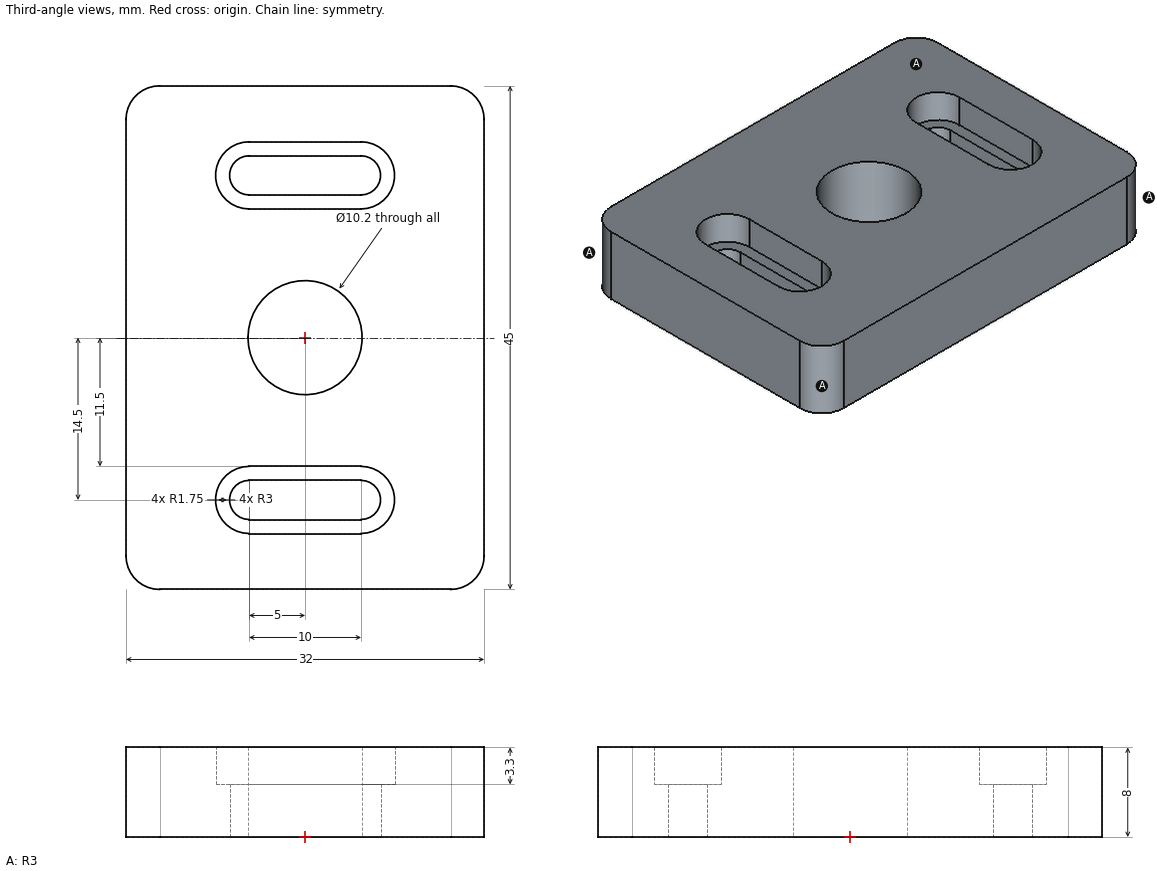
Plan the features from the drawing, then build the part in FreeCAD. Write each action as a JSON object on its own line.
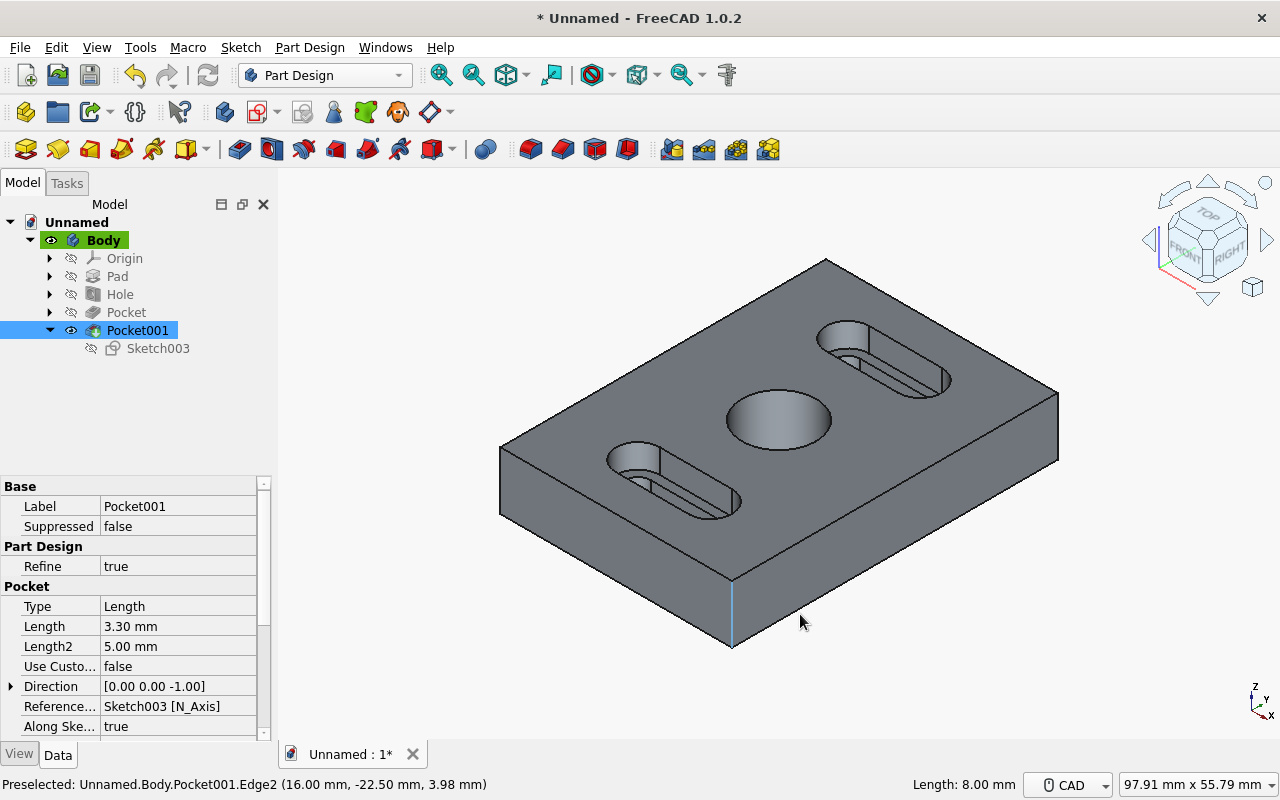
{"action": "key", "text": "2"}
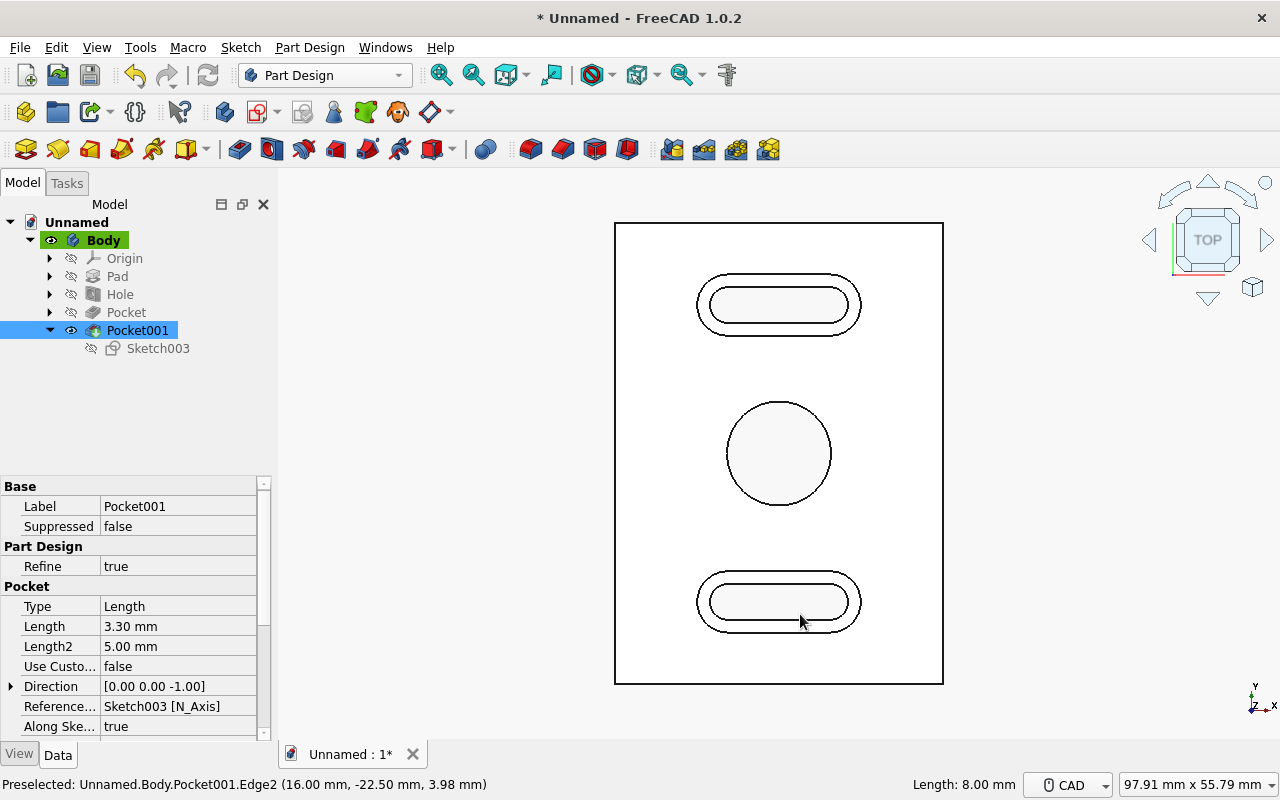
{"action": "key", "text": "1"}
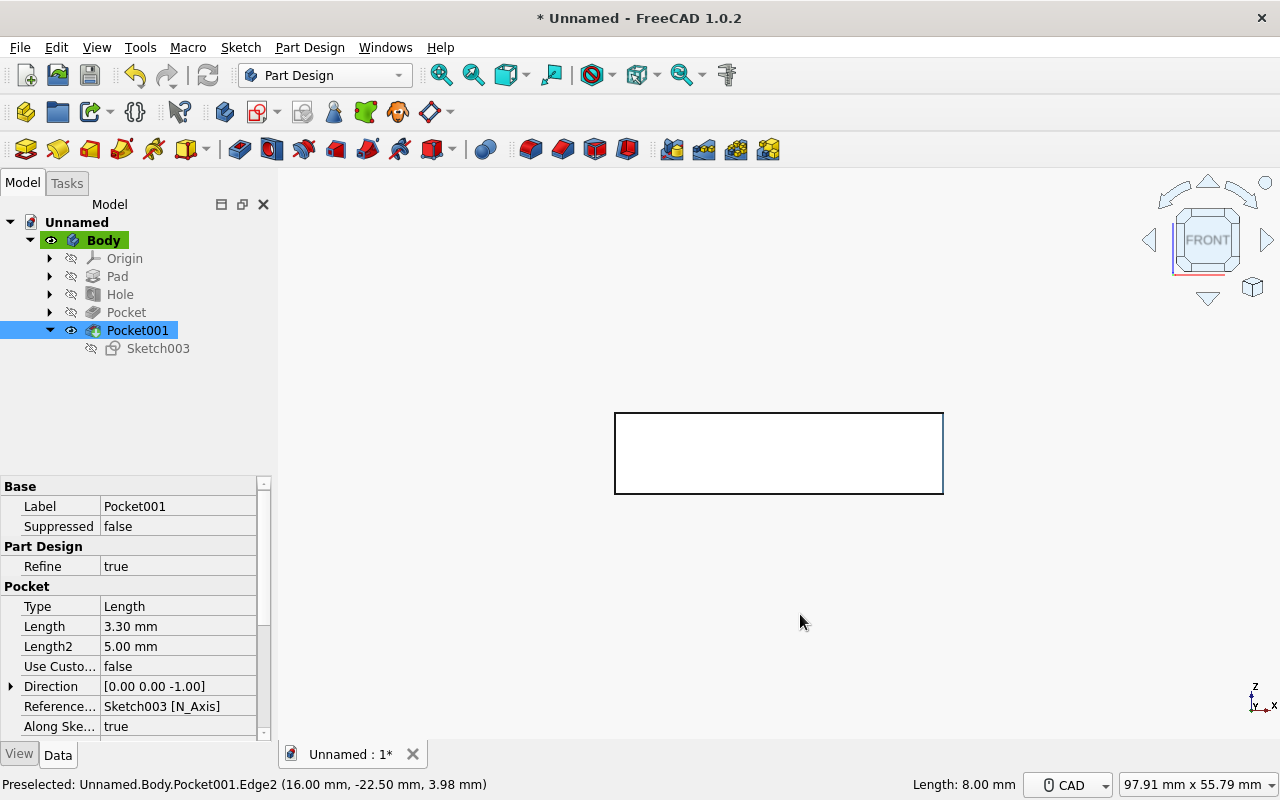
{"action": "left_click", "coordinate": [442, 76]}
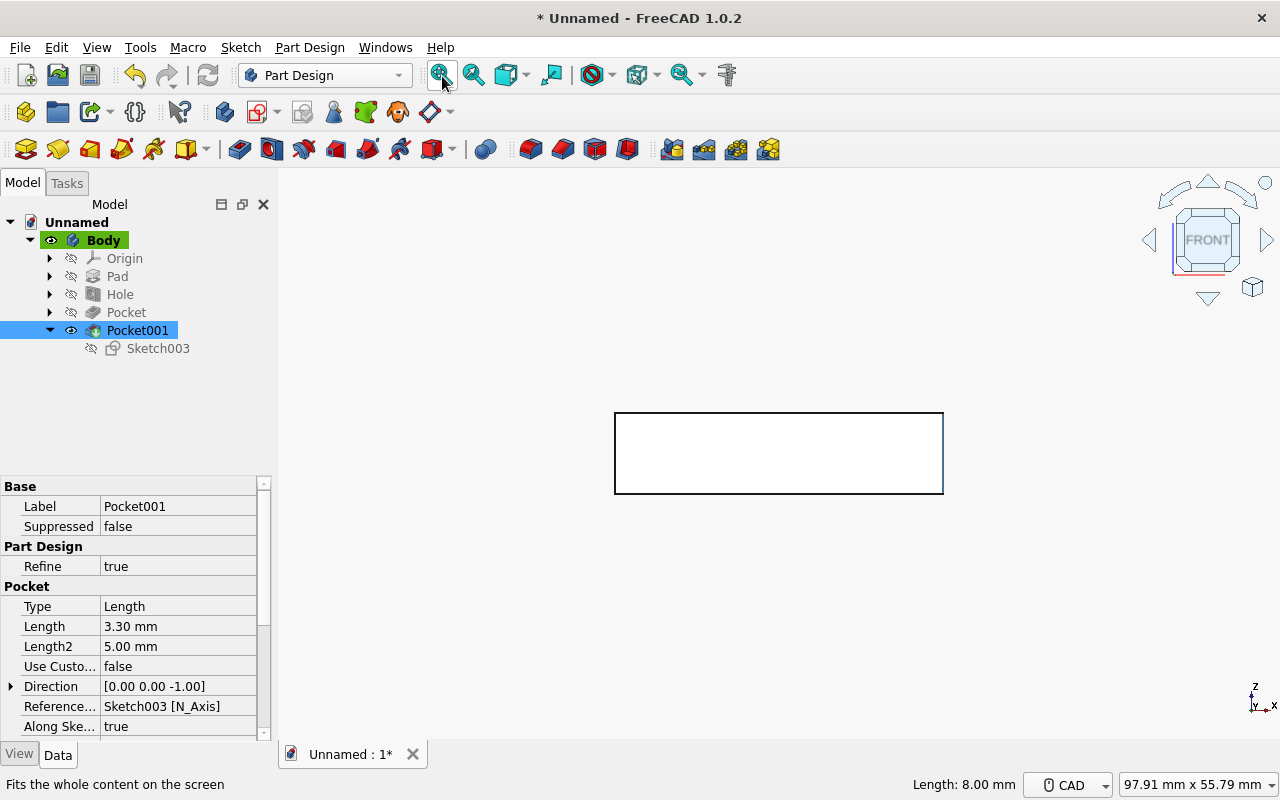
{"action": "left_click", "coordinate": [615, 453], "text": "ctrl"}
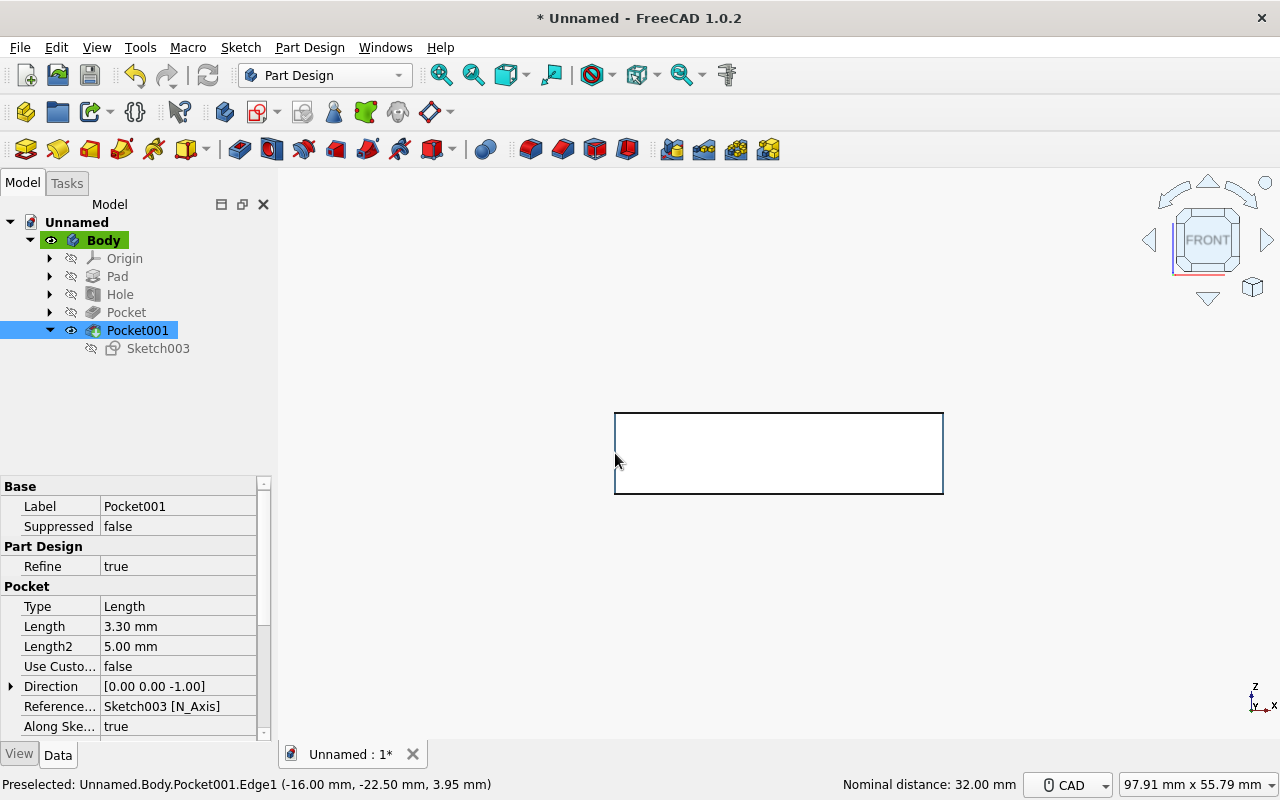
{"action": "key", "text": "3"}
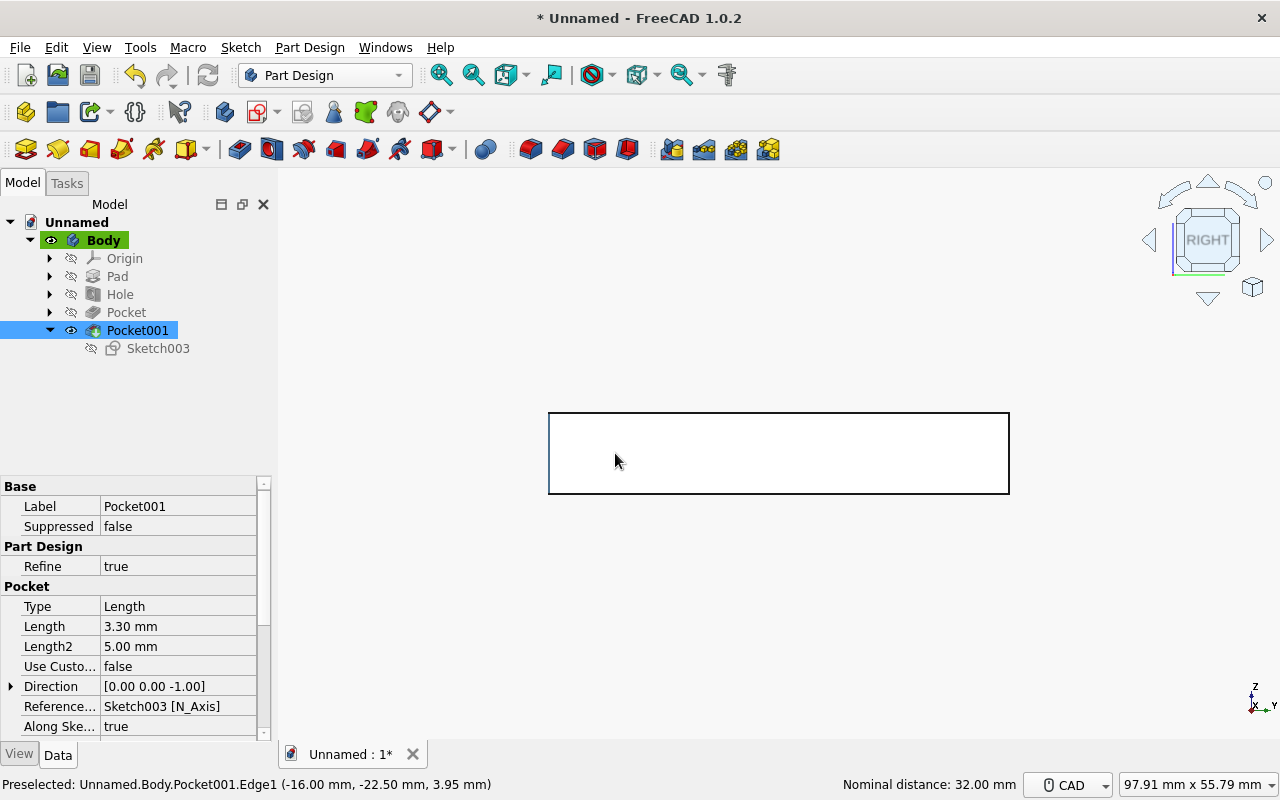
{"action": "left_click", "coordinate": [1009, 452], "text": "ctrl"}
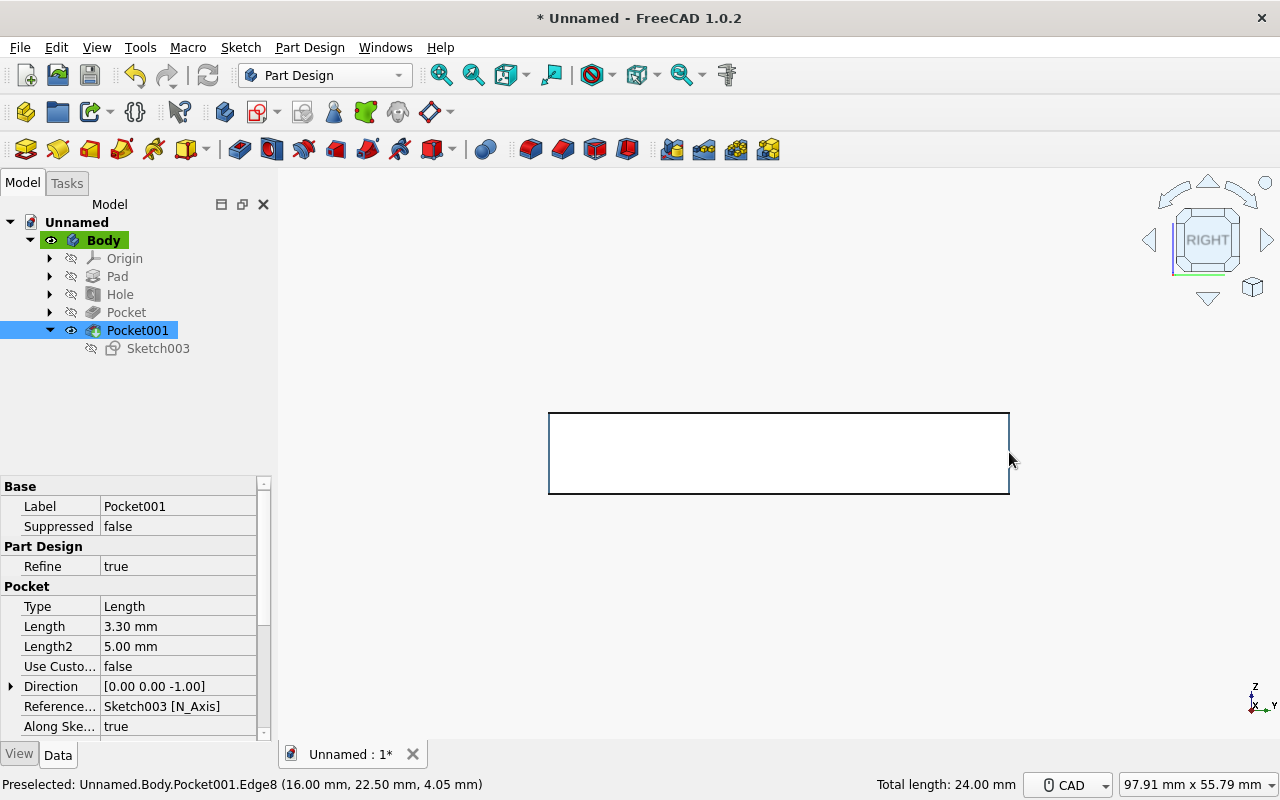
{"action": "key", "text": "5"}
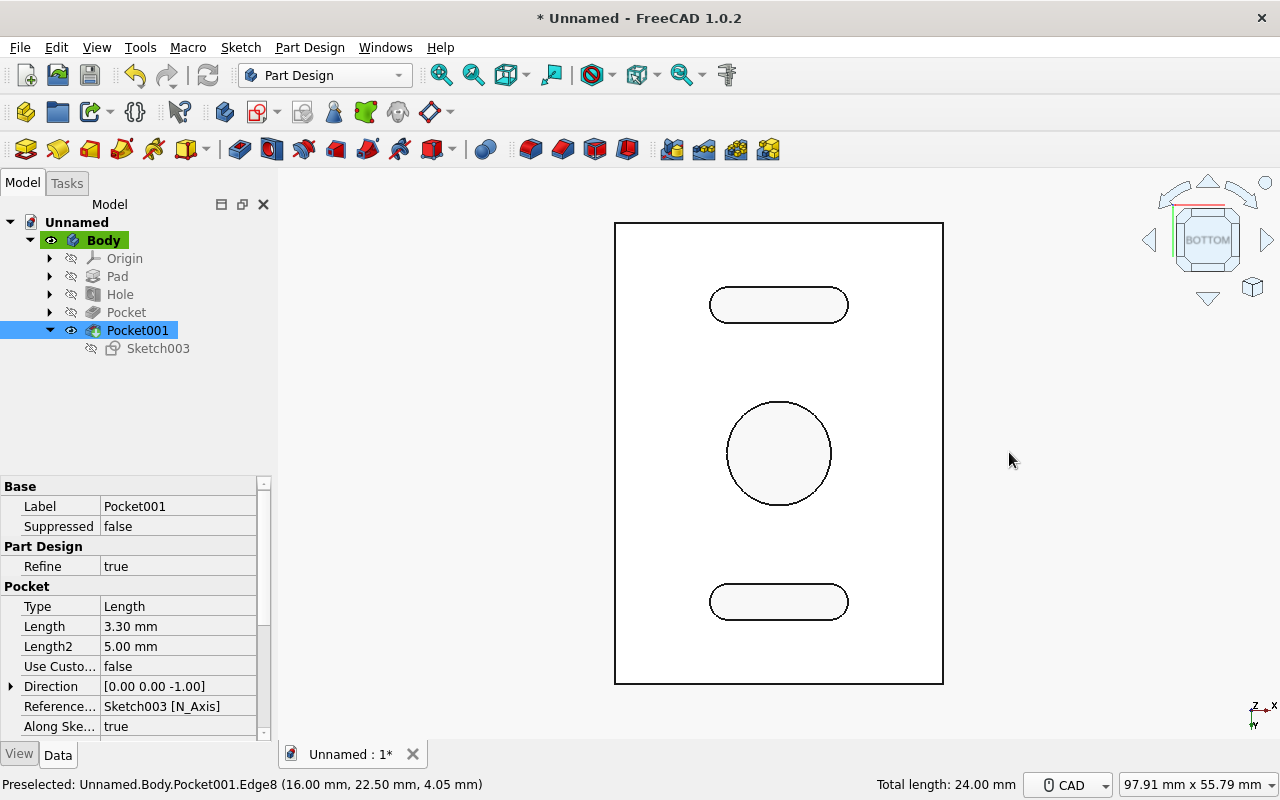
{"action": "key", "text": "4"}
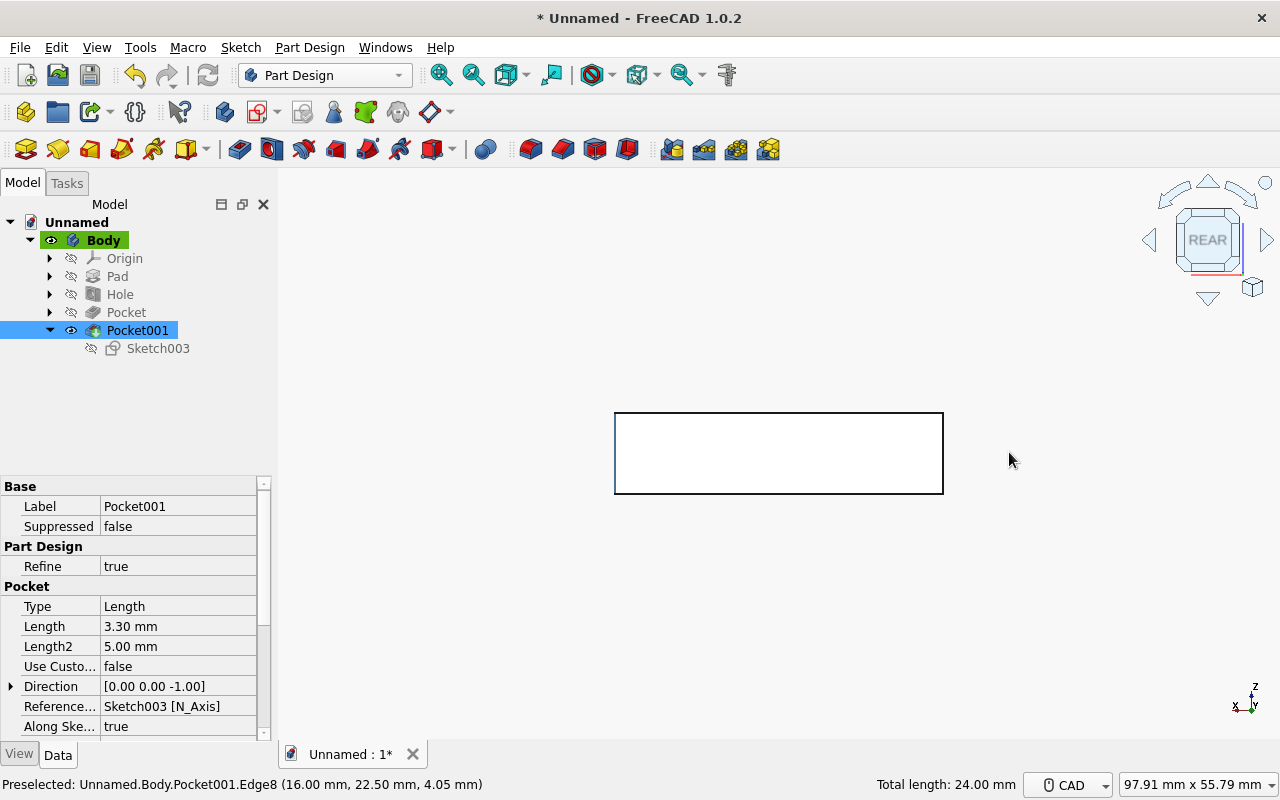
{"action": "left_click", "coordinate": [442, 76]}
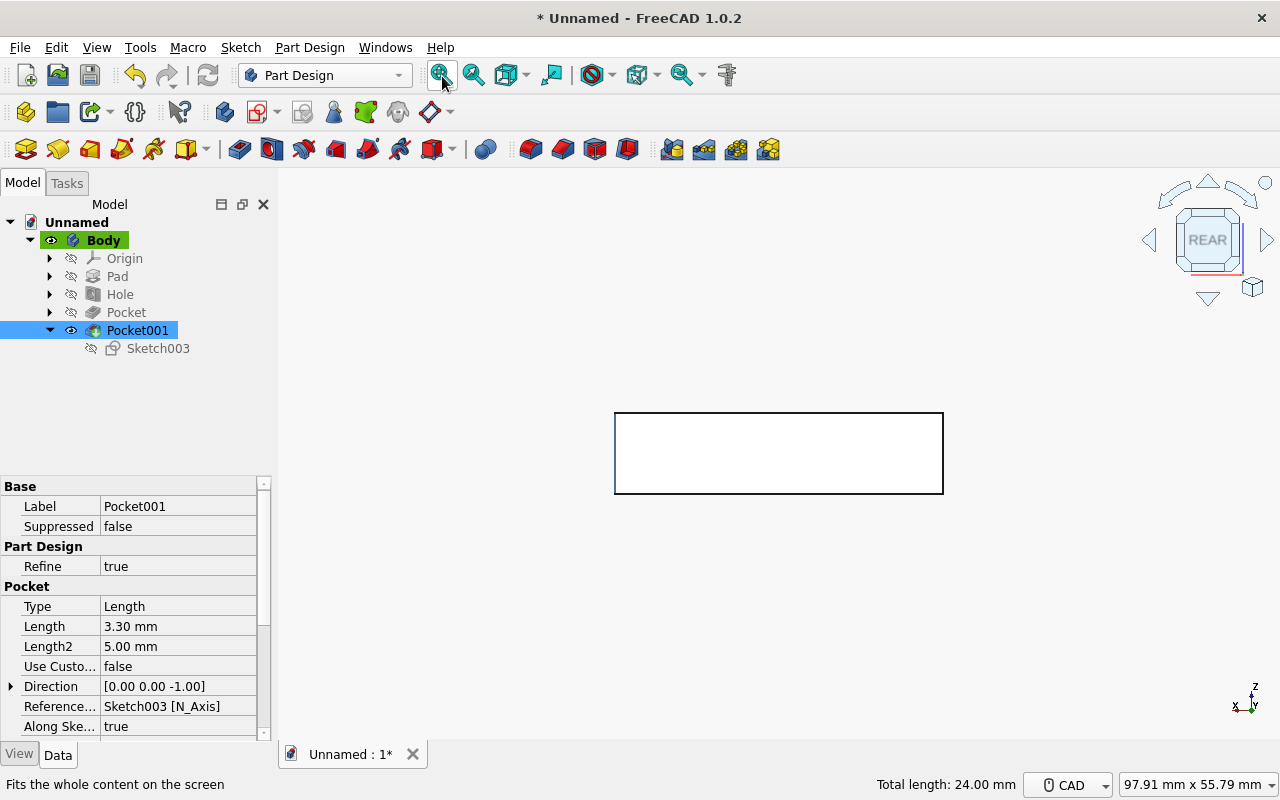
{"action": "left_click", "coordinate": [943, 453], "text": "ctrl"}